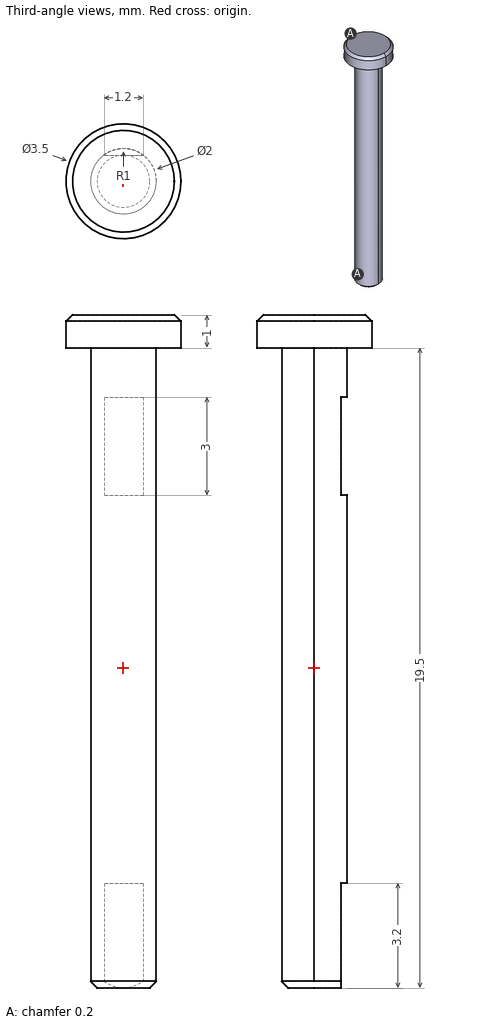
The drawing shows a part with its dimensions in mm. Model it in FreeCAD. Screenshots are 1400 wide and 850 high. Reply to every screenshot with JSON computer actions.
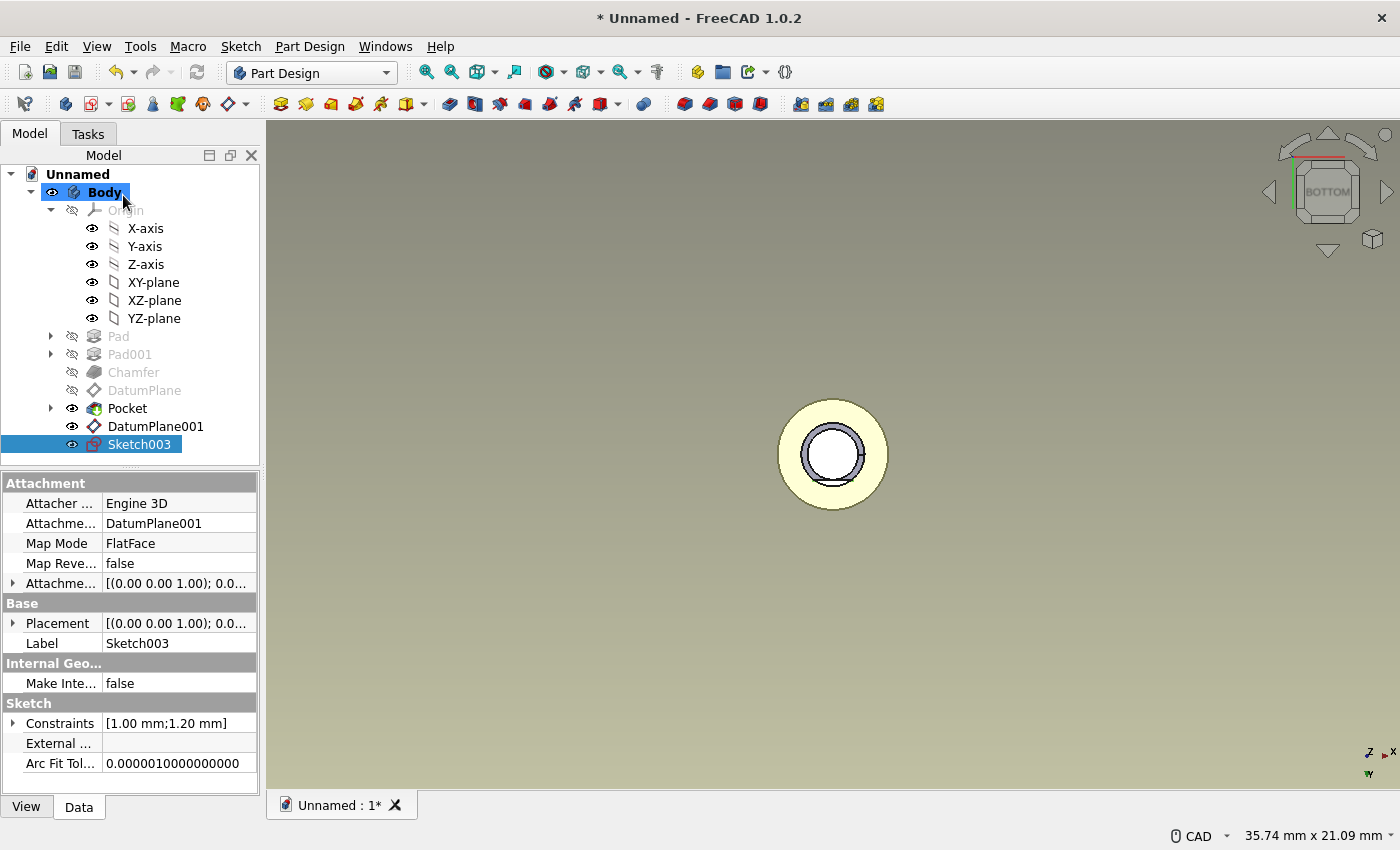
{"action": "left_click", "coordinate": [450, 104]}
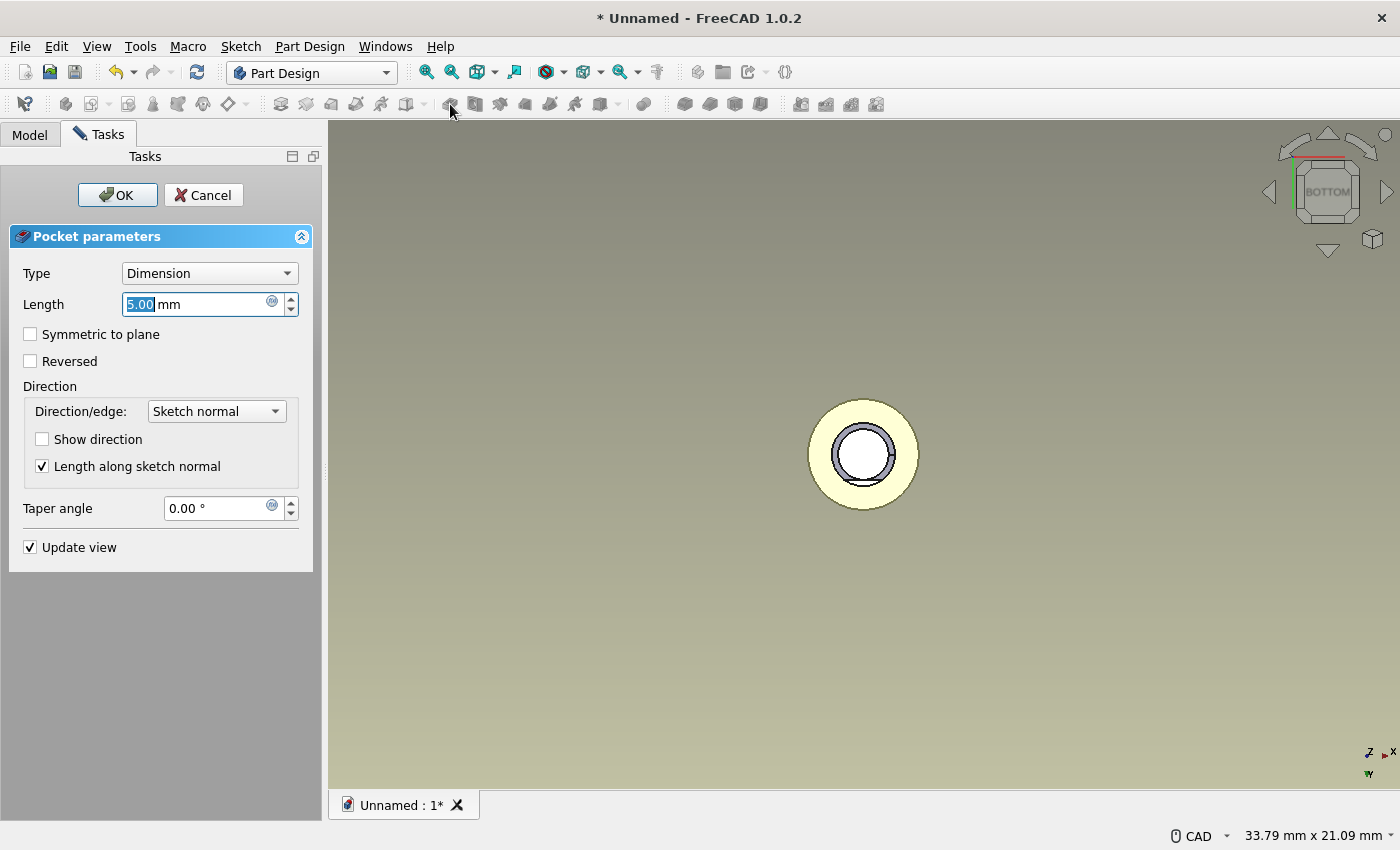
{"action": "type", "text": "3"}
{"action": "key", "text": "Tab"}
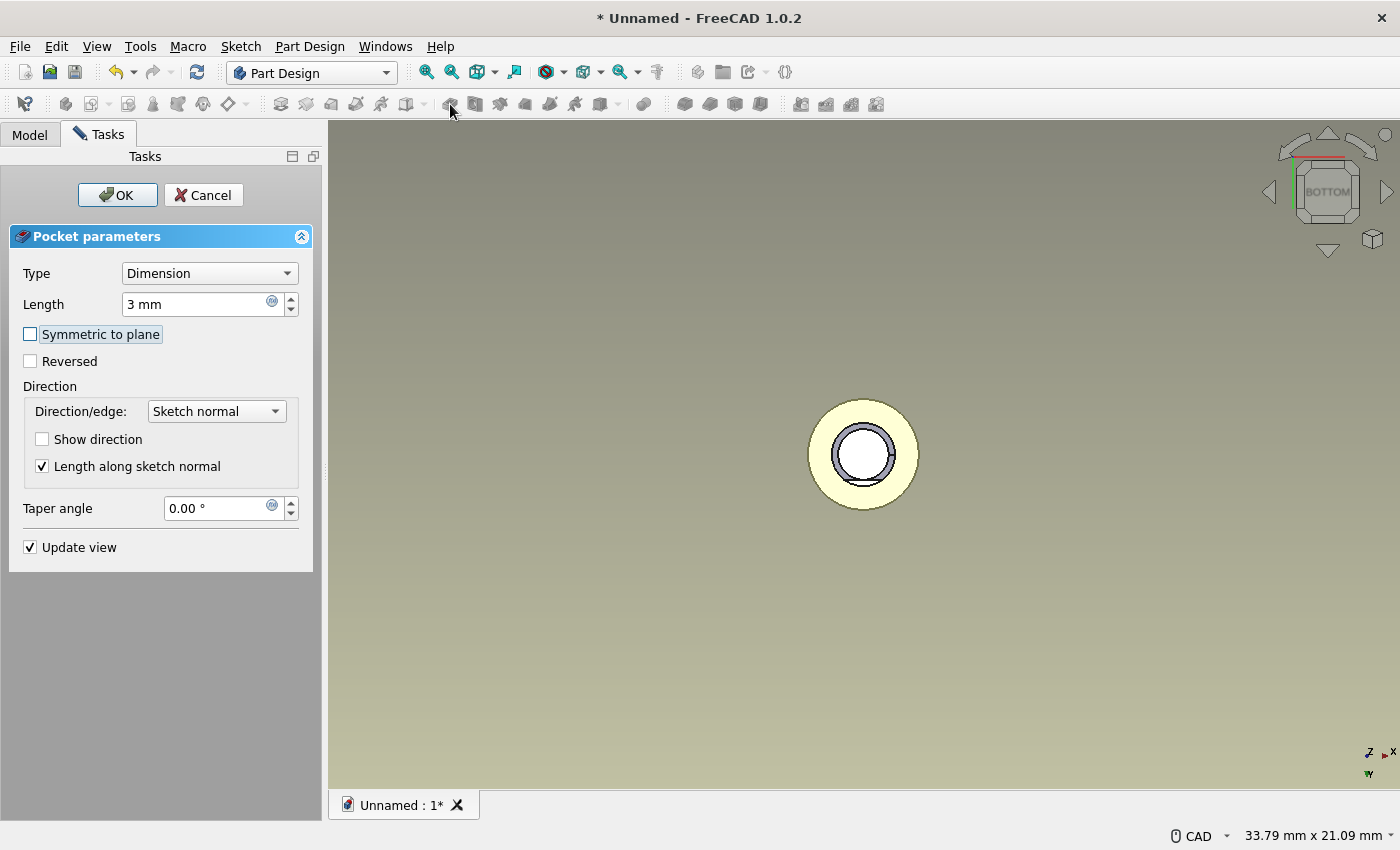
{"action": "left_click", "coordinate": [31, 334]}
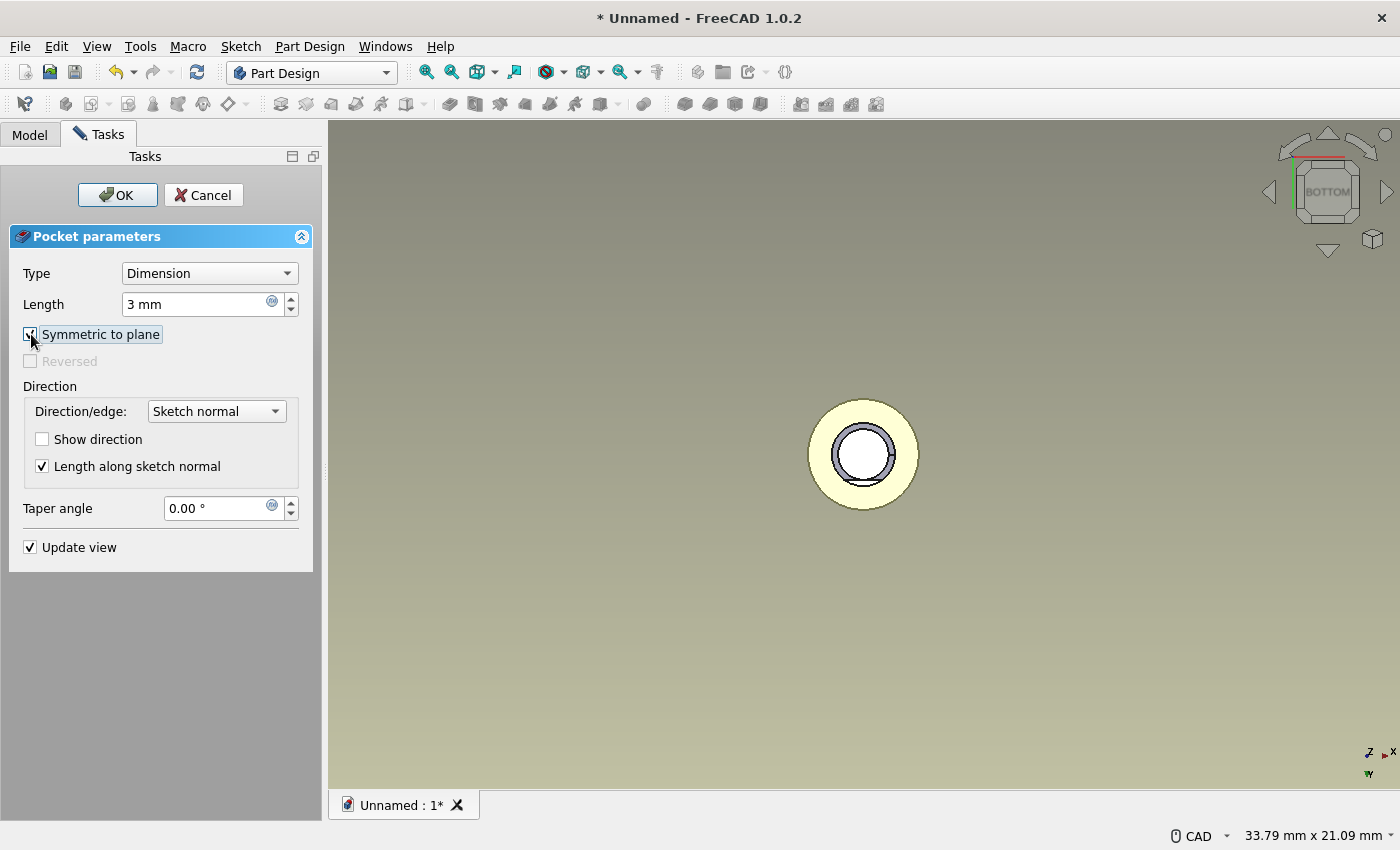
{"action": "left_click", "coordinate": [118, 195]}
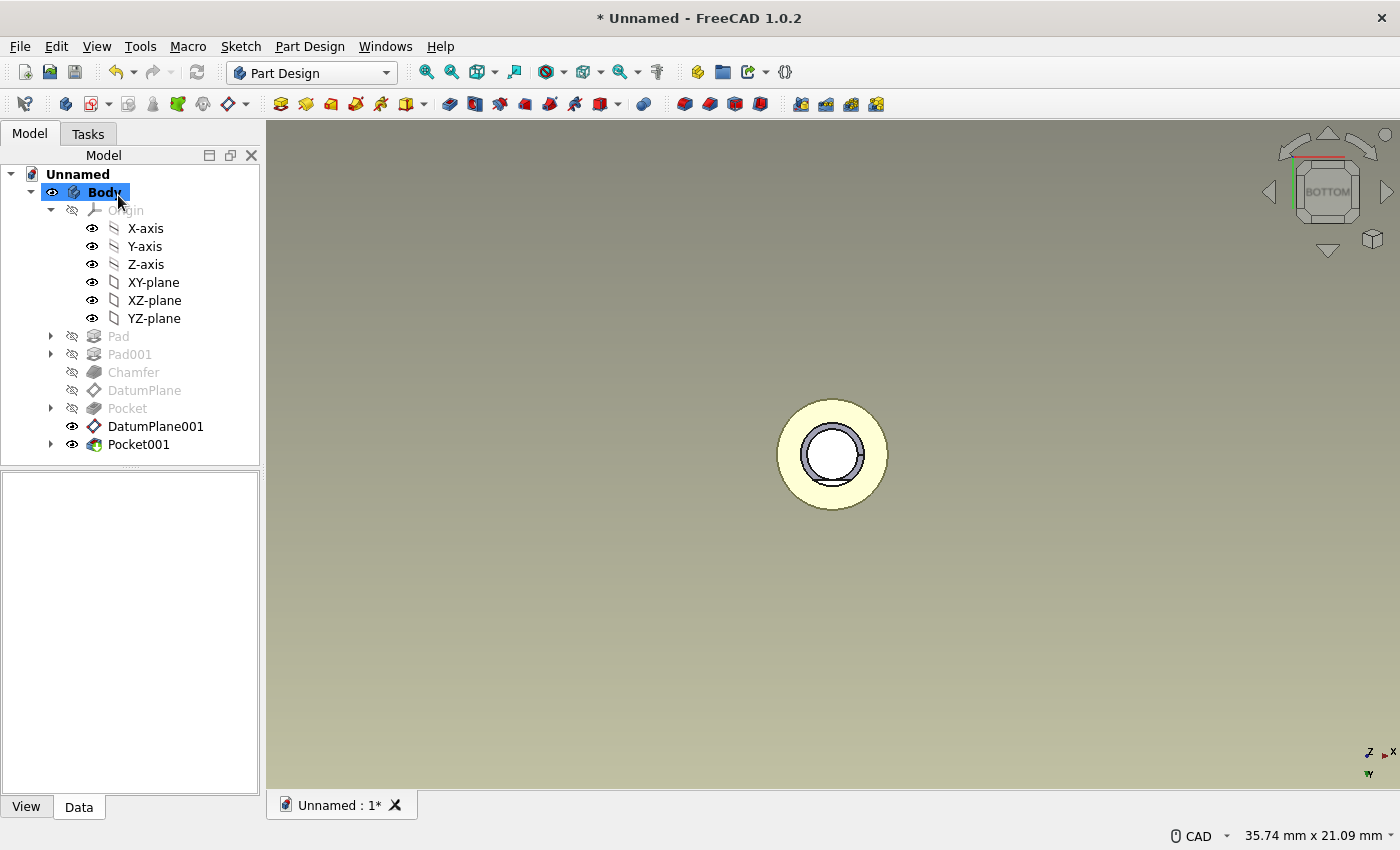
{"action": "left_click", "coordinate": [117, 426]}
{"action": "key", "text": "space"}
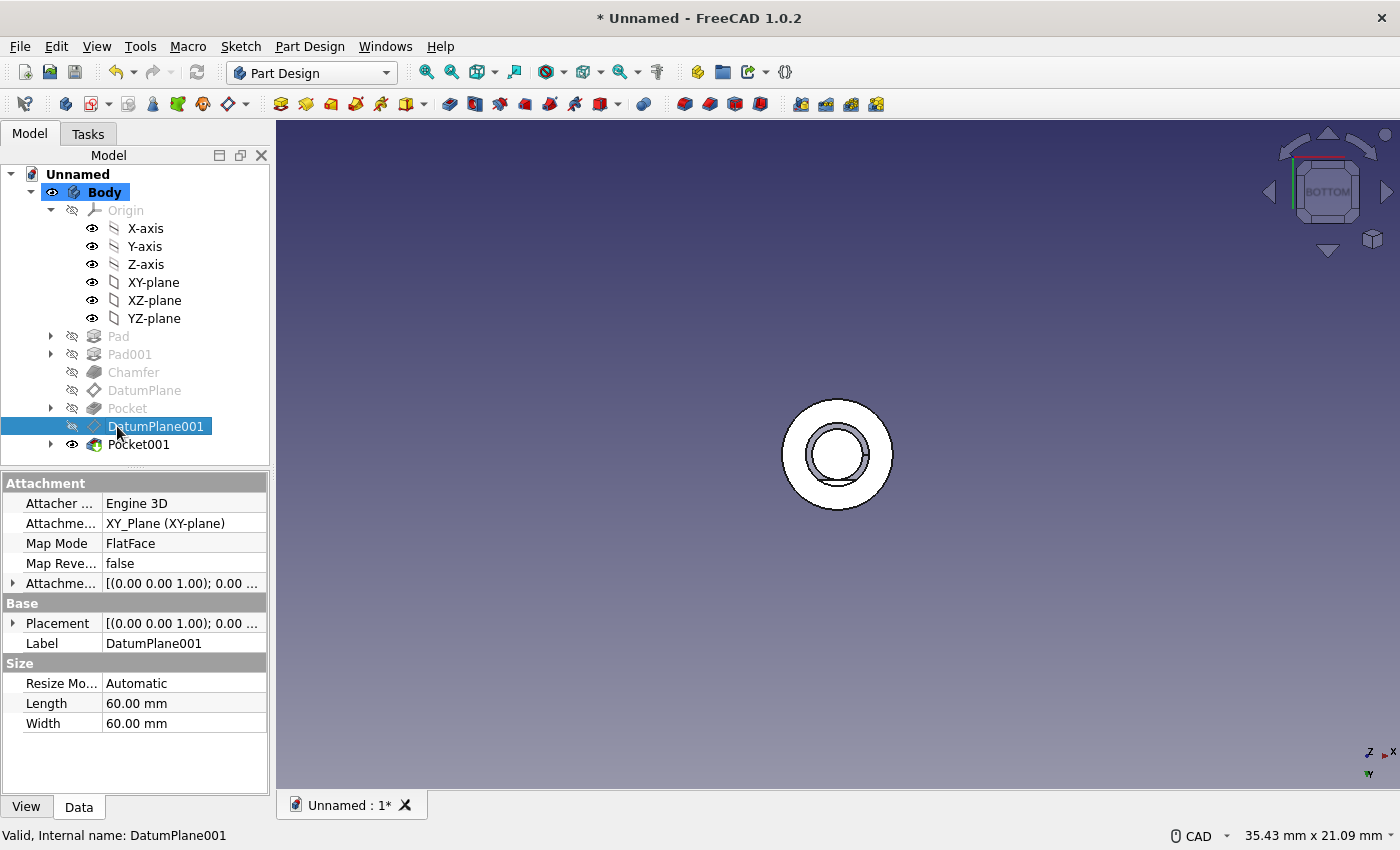
{"action": "key", "text": "0"}